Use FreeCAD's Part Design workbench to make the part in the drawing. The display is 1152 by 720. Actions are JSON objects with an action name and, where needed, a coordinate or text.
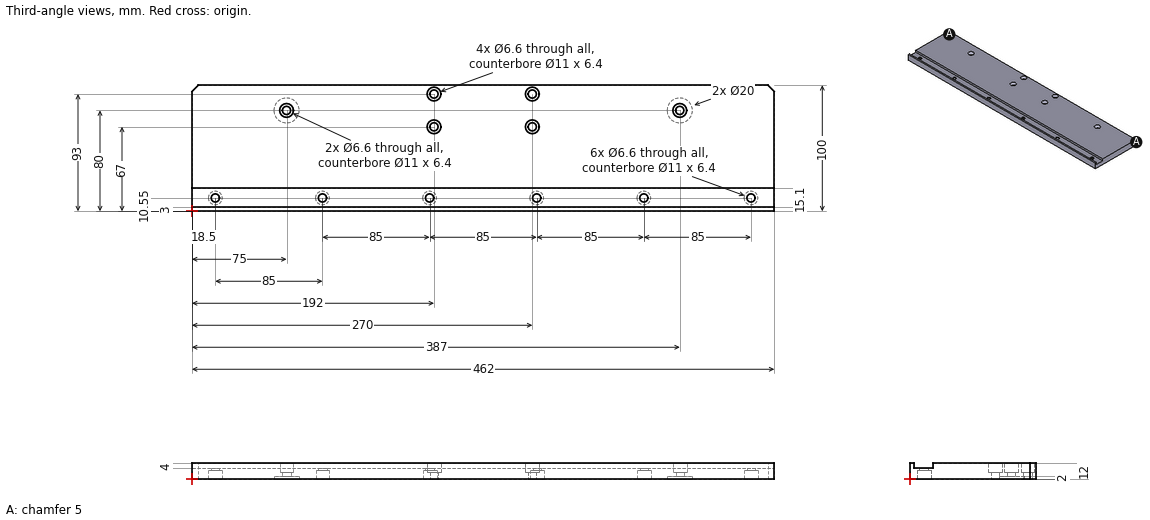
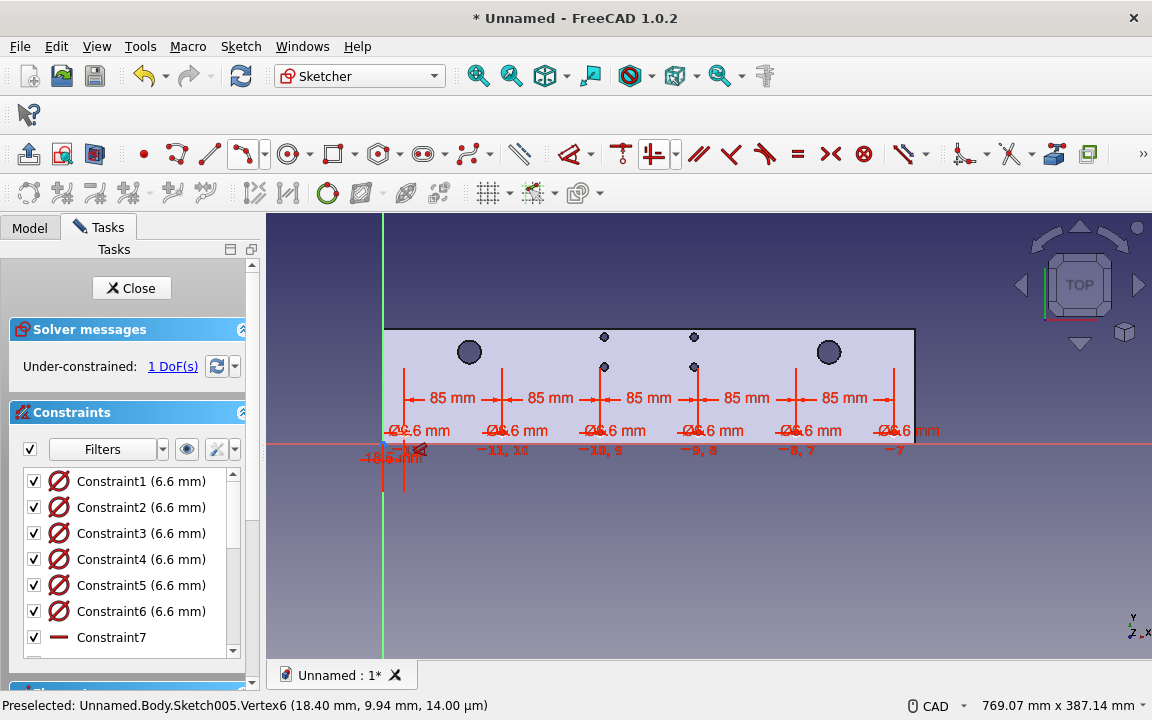
{"action": "scroll", "coordinate": [894, 433], "scroll_direction": "up", "scroll_amount": 6}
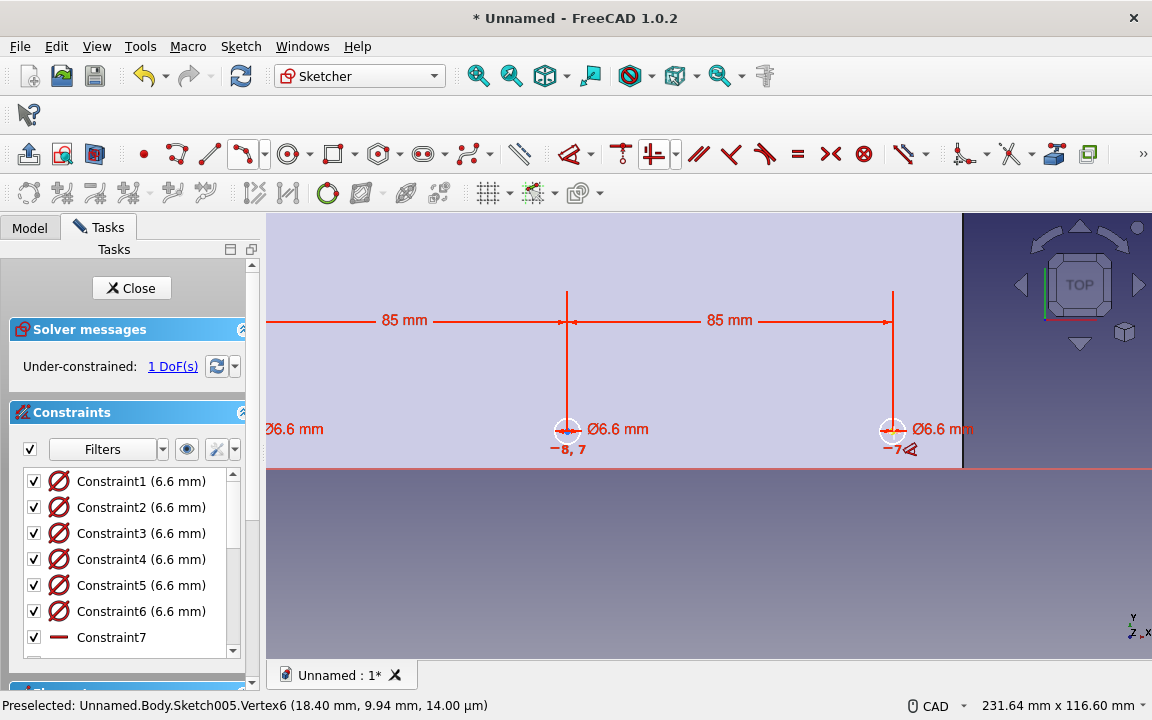
{"action": "left_click", "coordinate": [893, 431]}
{"action": "left_click", "coordinate": [927, 450]}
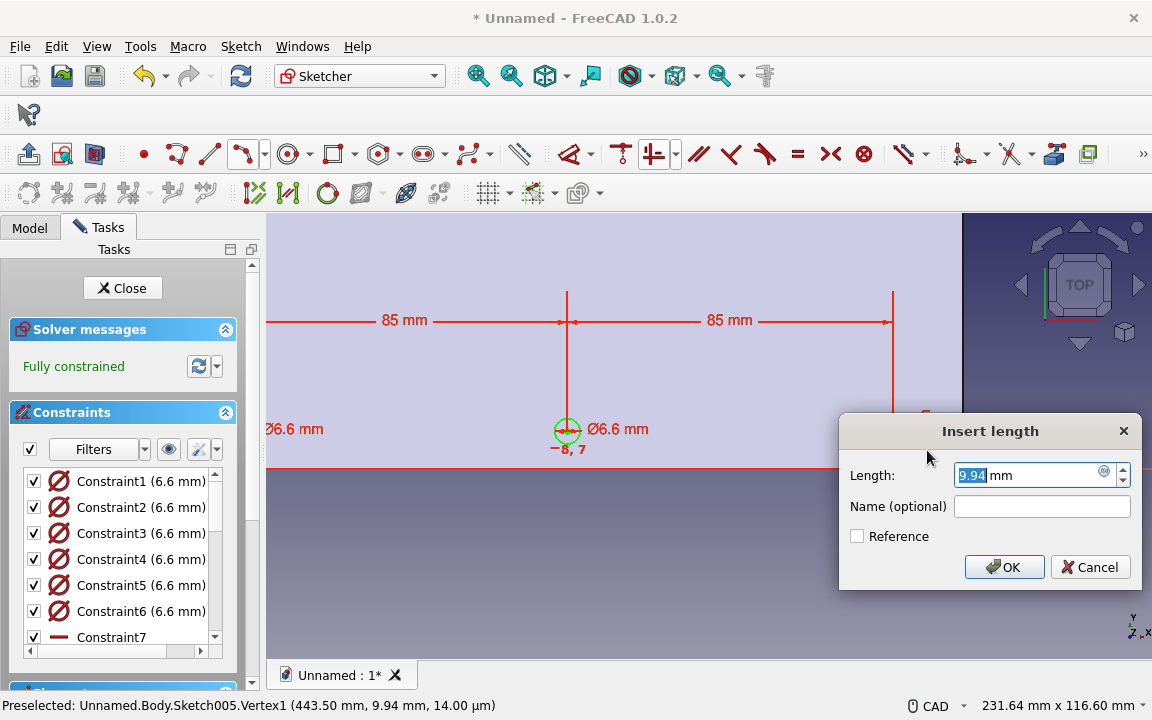
{"action": "type", "text": "10.55"}
{"action": "key", "text": "Return"}
{"action": "key", "text": "Escape"}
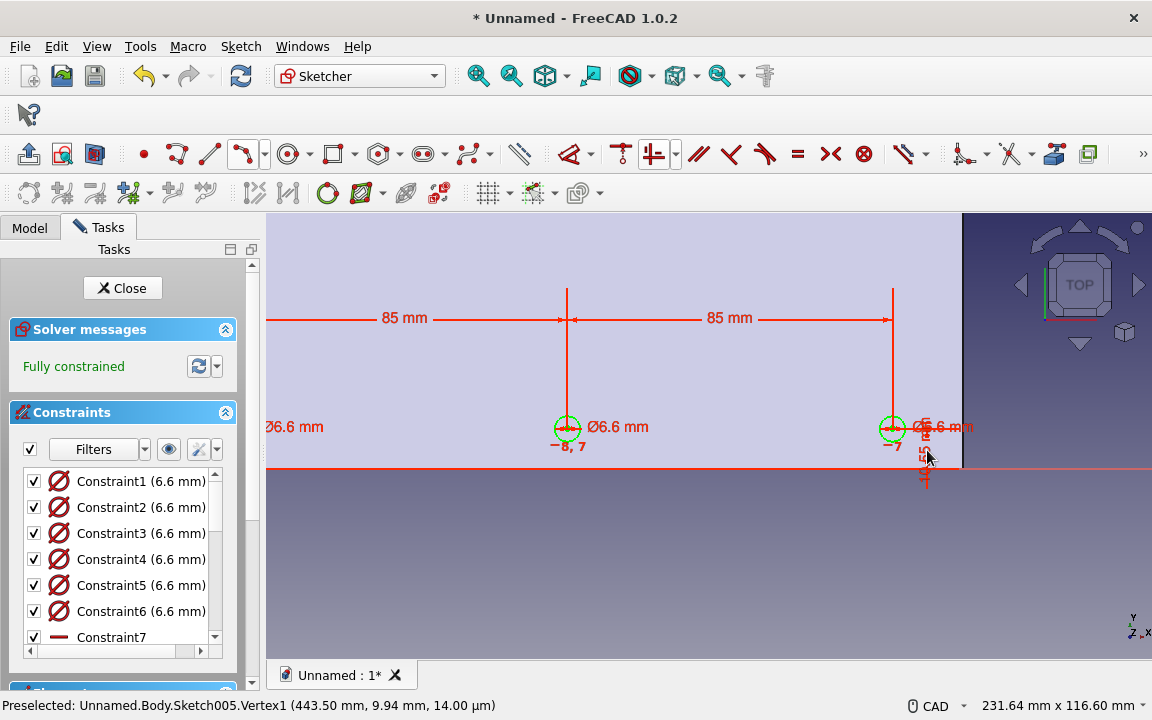
{"action": "left_click", "coordinate": [123, 288]}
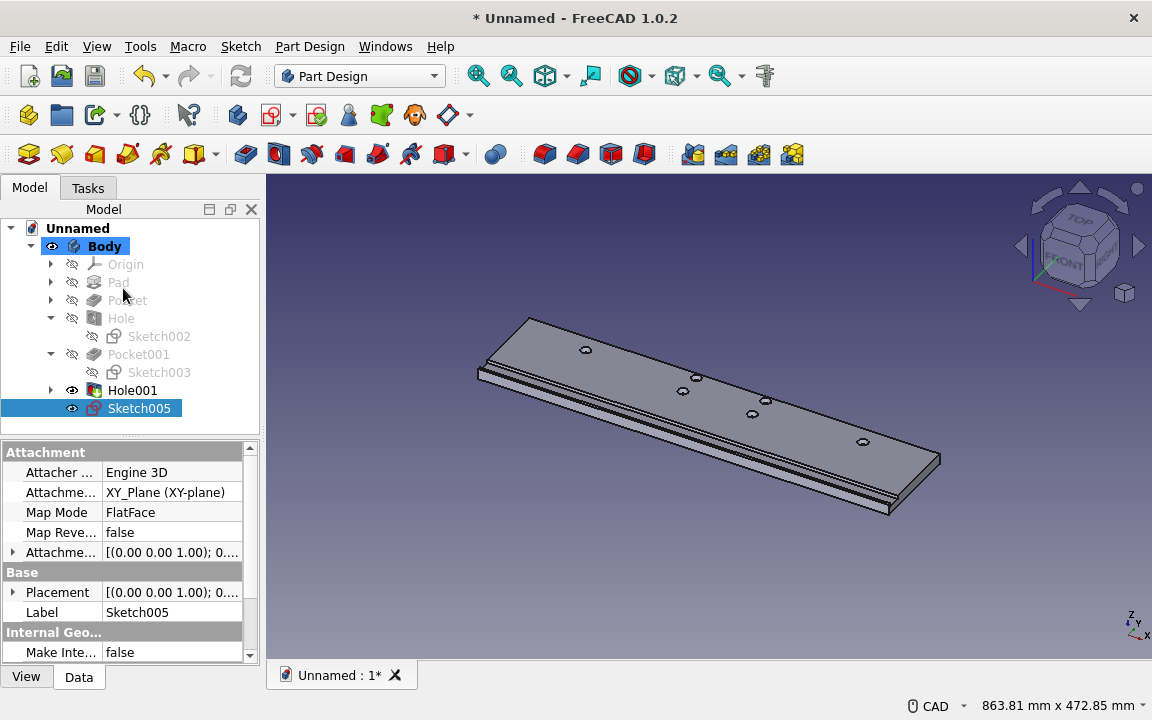
{"action": "left_click", "coordinate": [279, 154]}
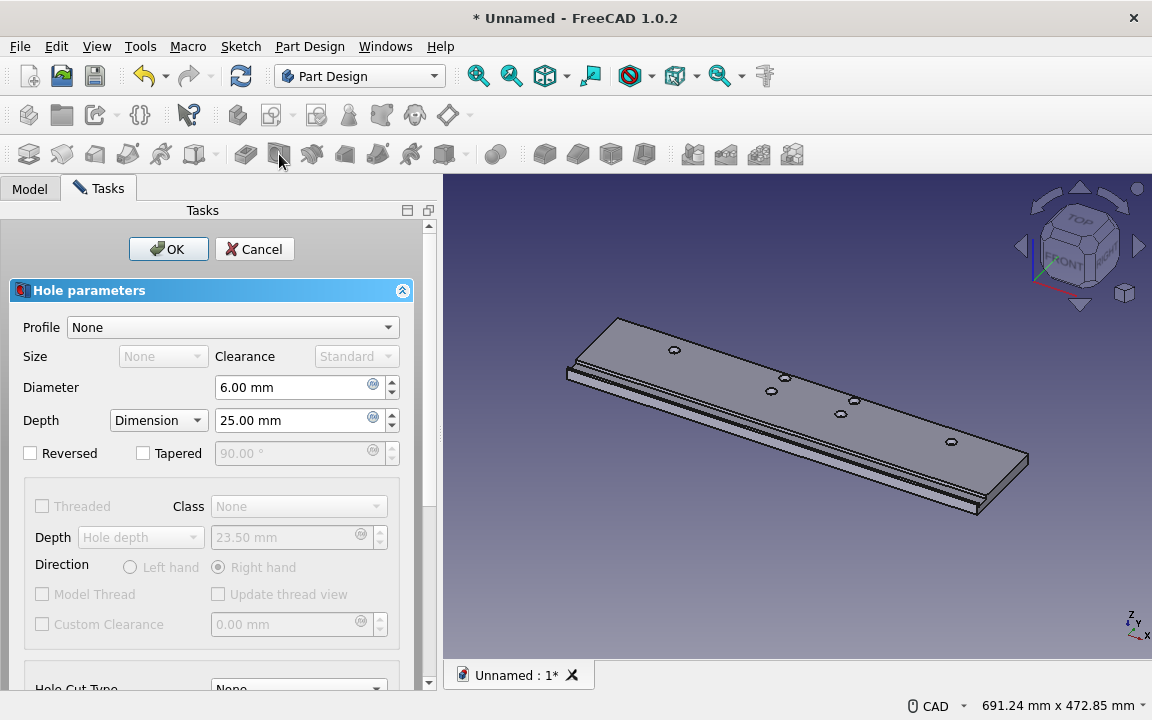
{"action": "triple_click", "coordinate": [300, 388]}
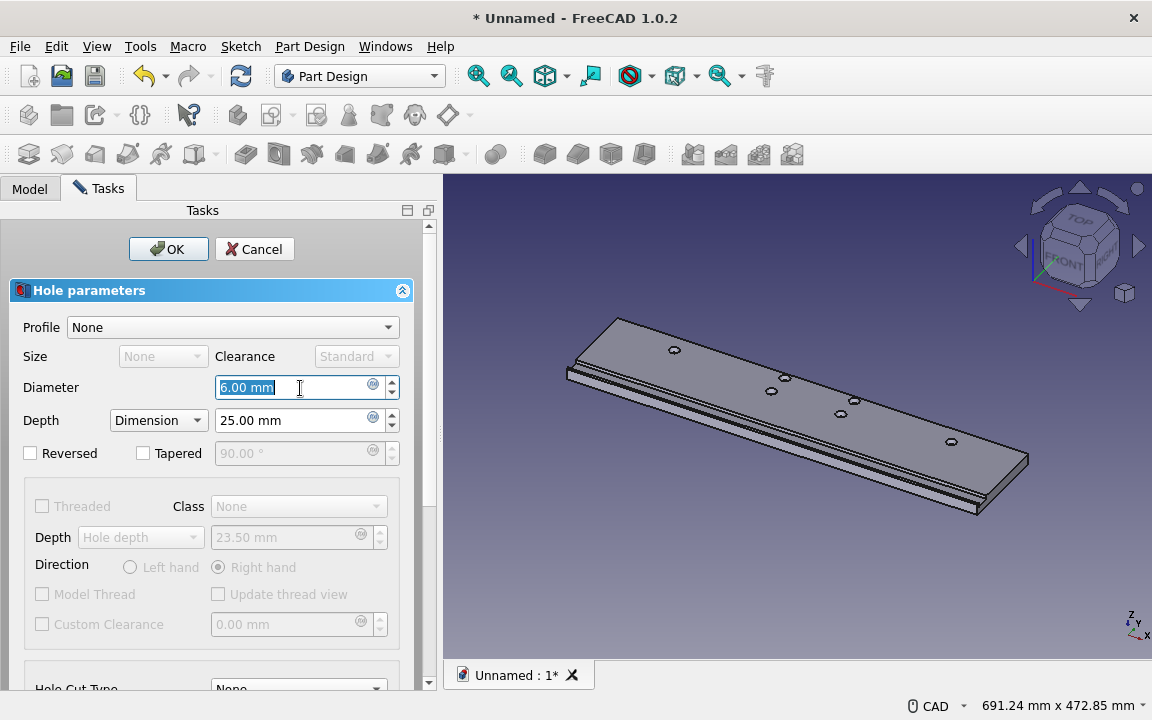
{"action": "type", "text": "6.6"}
{"action": "key", "text": "Tab"}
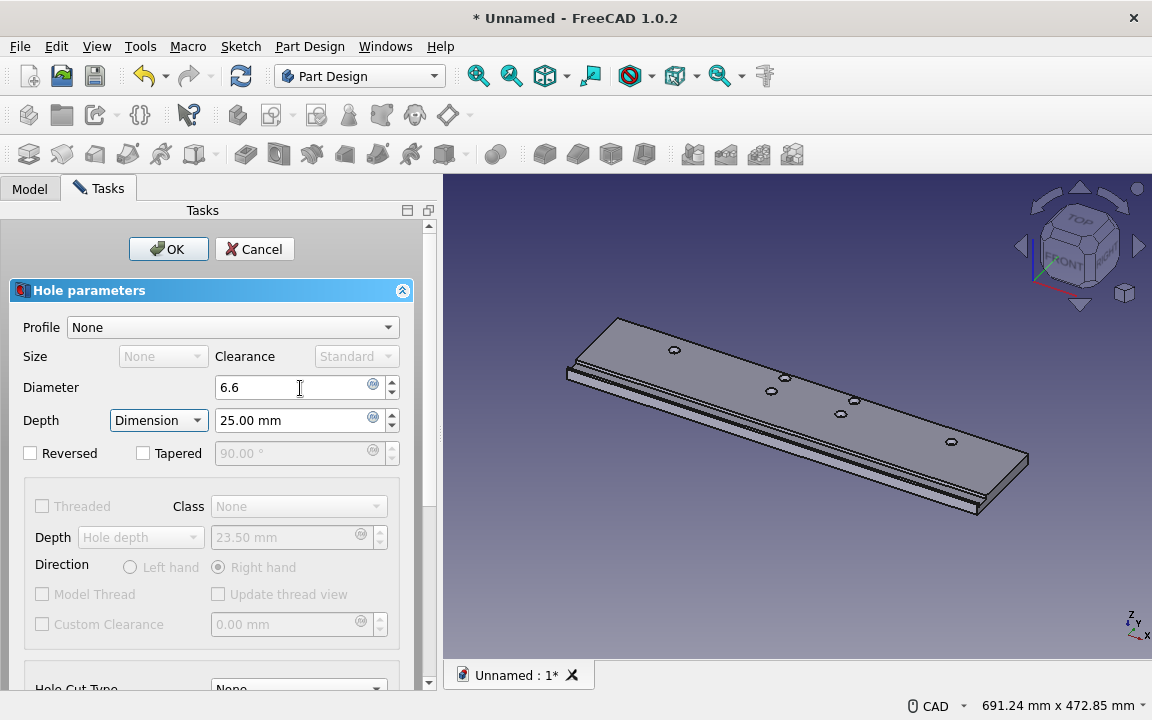
{"action": "left_click", "coordinate": [160, 420]}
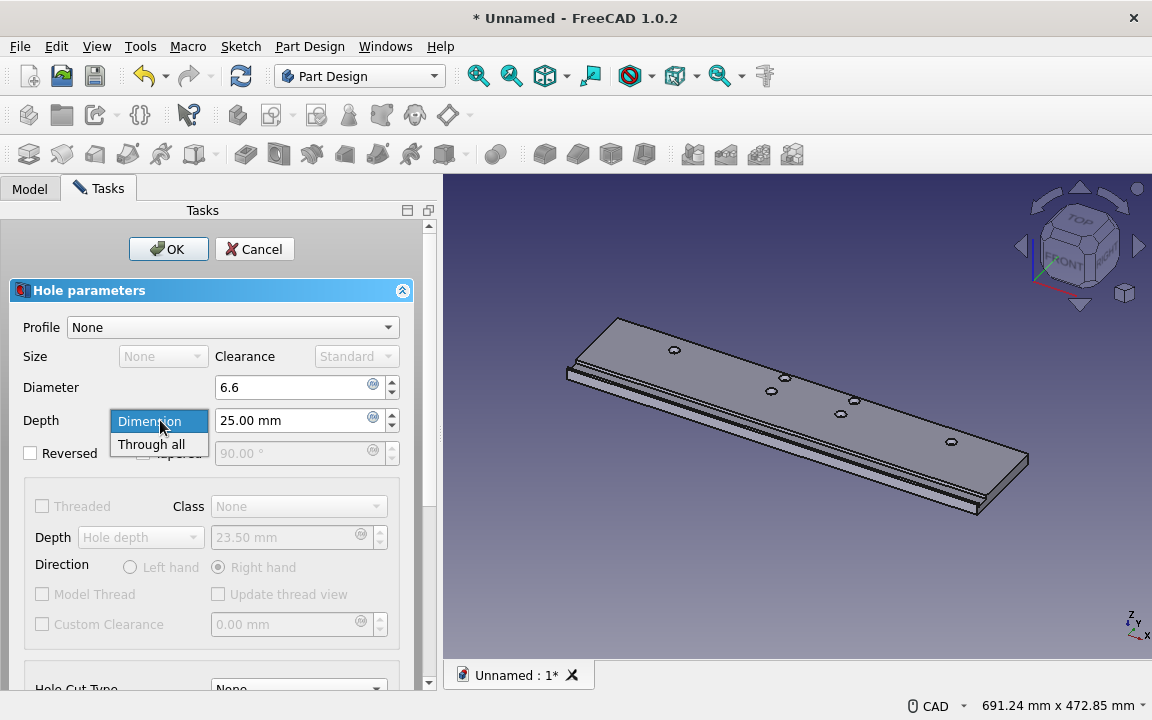
{"action": "left_click", "coordinate": [158, 444]}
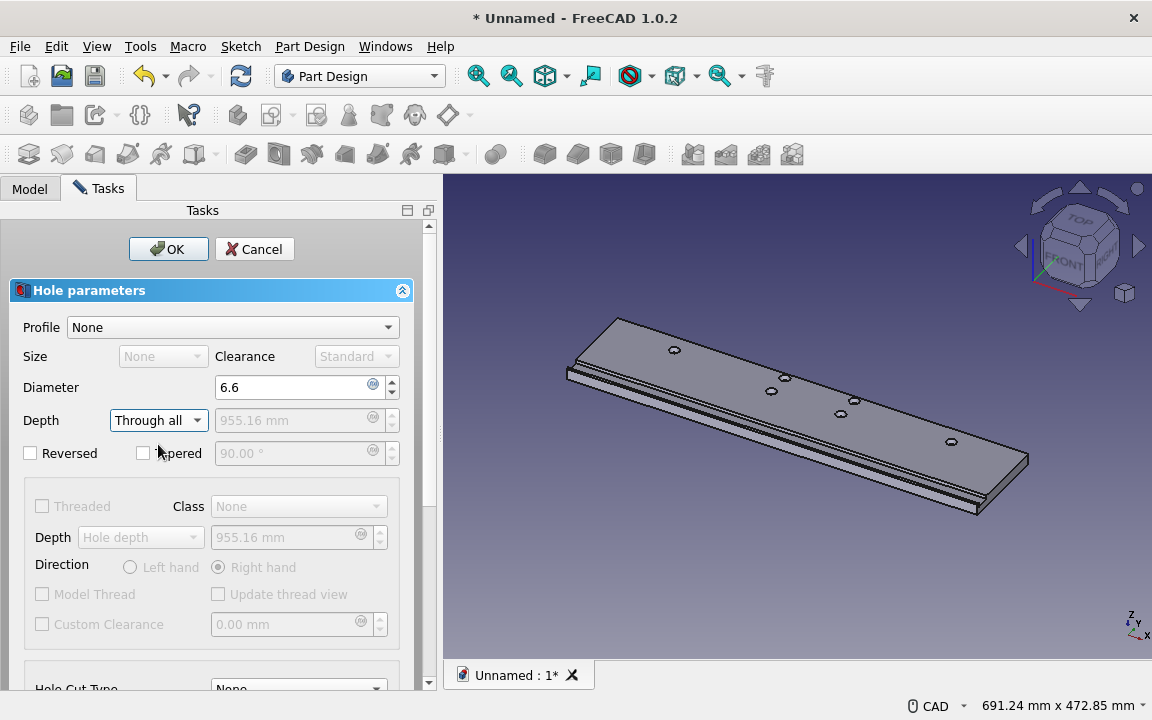
{"action": "left_click", "coordinate": [31, 453]}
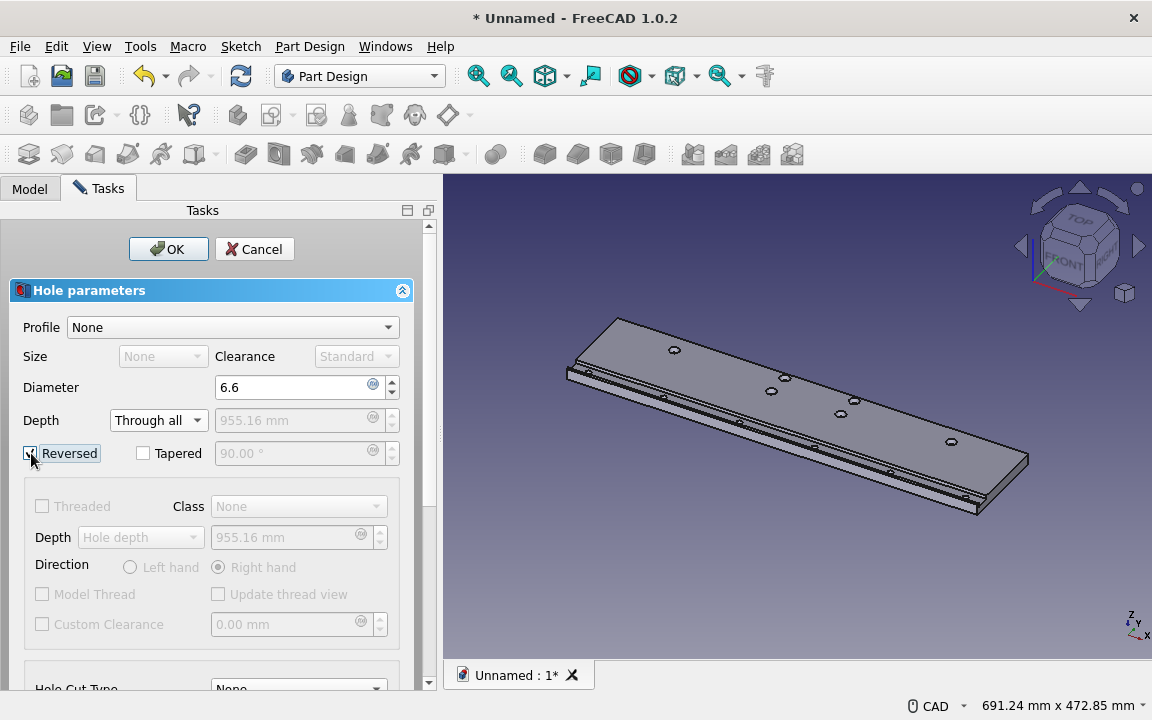
{"action": "scroll", "coordinate": [429, 455], "scroll_direction": "down", "scroll_amount": 2}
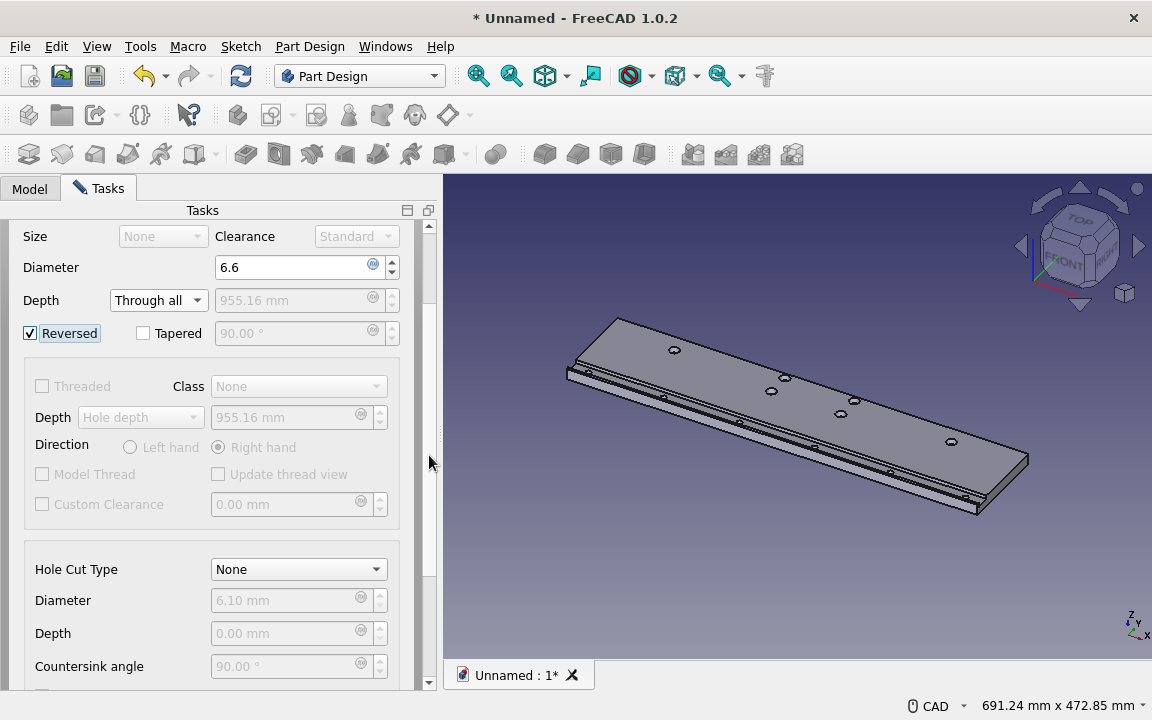
{"action": "left_click", "coordinate": [300, 570]}